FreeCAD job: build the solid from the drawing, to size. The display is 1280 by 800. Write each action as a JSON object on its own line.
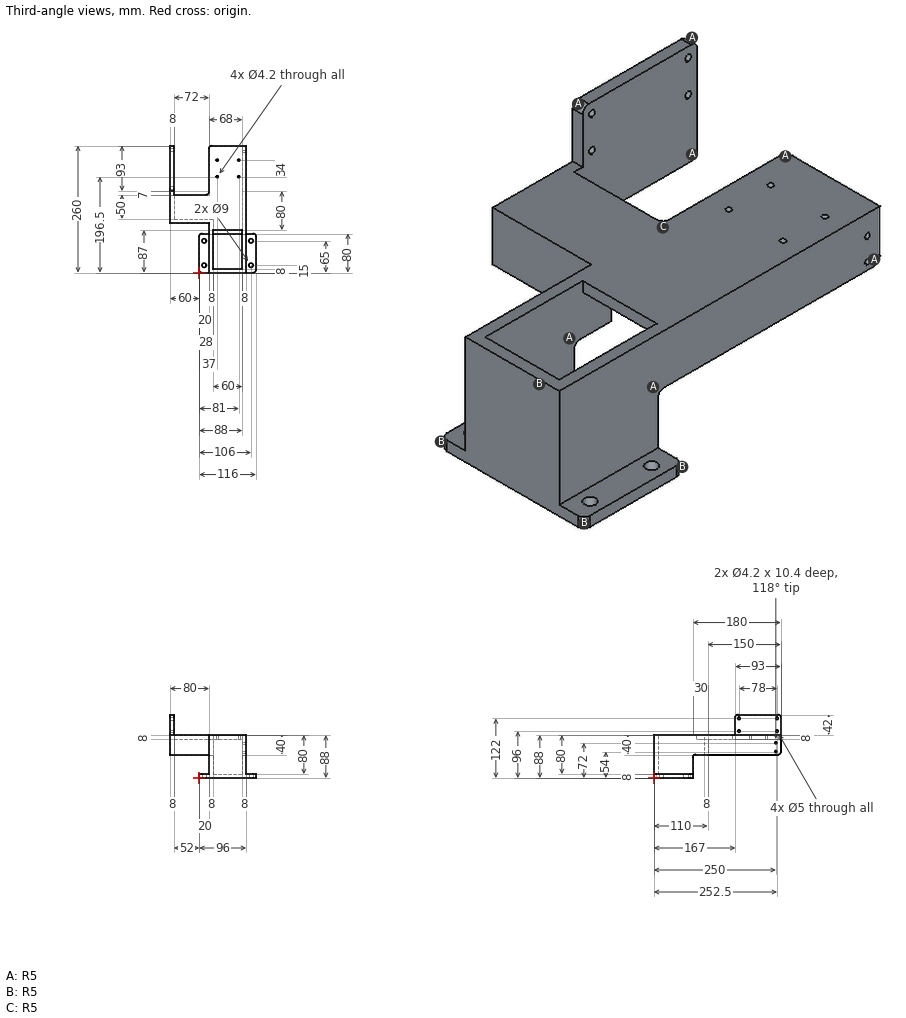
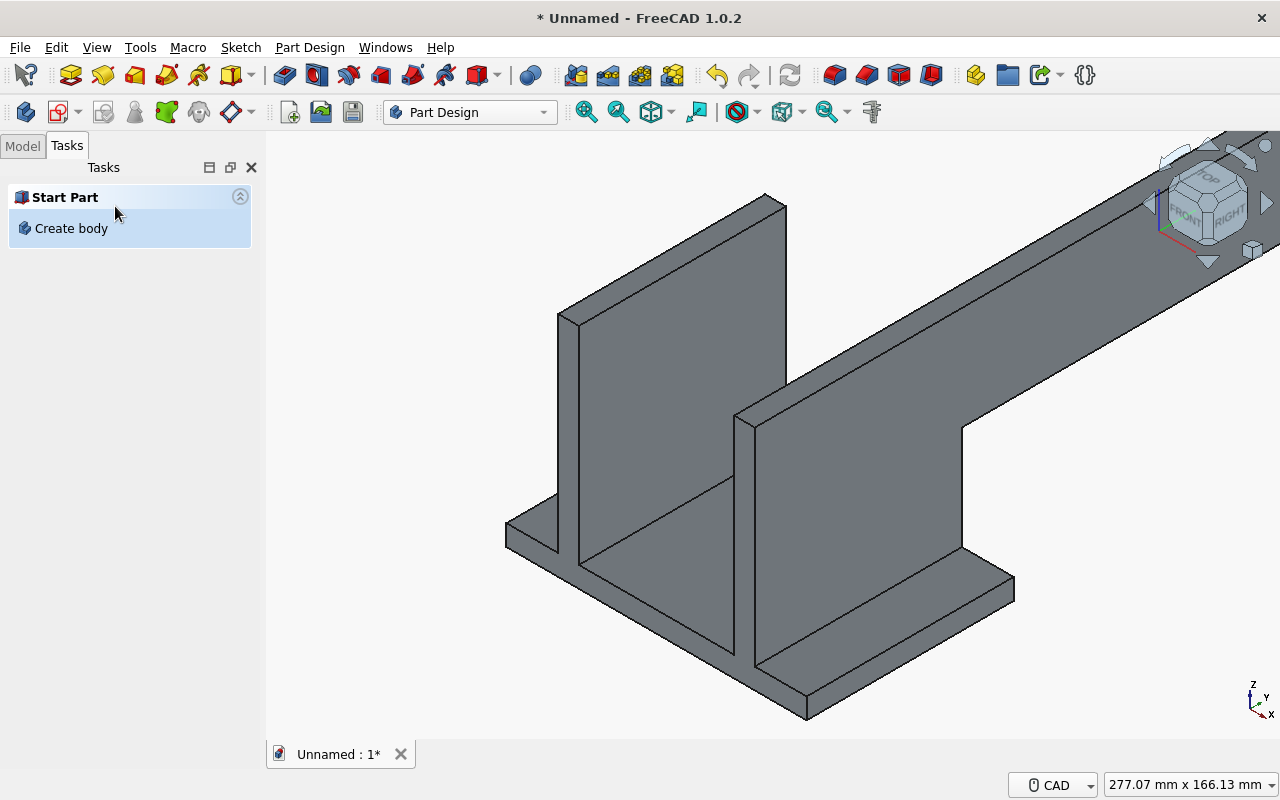
{"action": "left_click", "coordinate": [588, 112]}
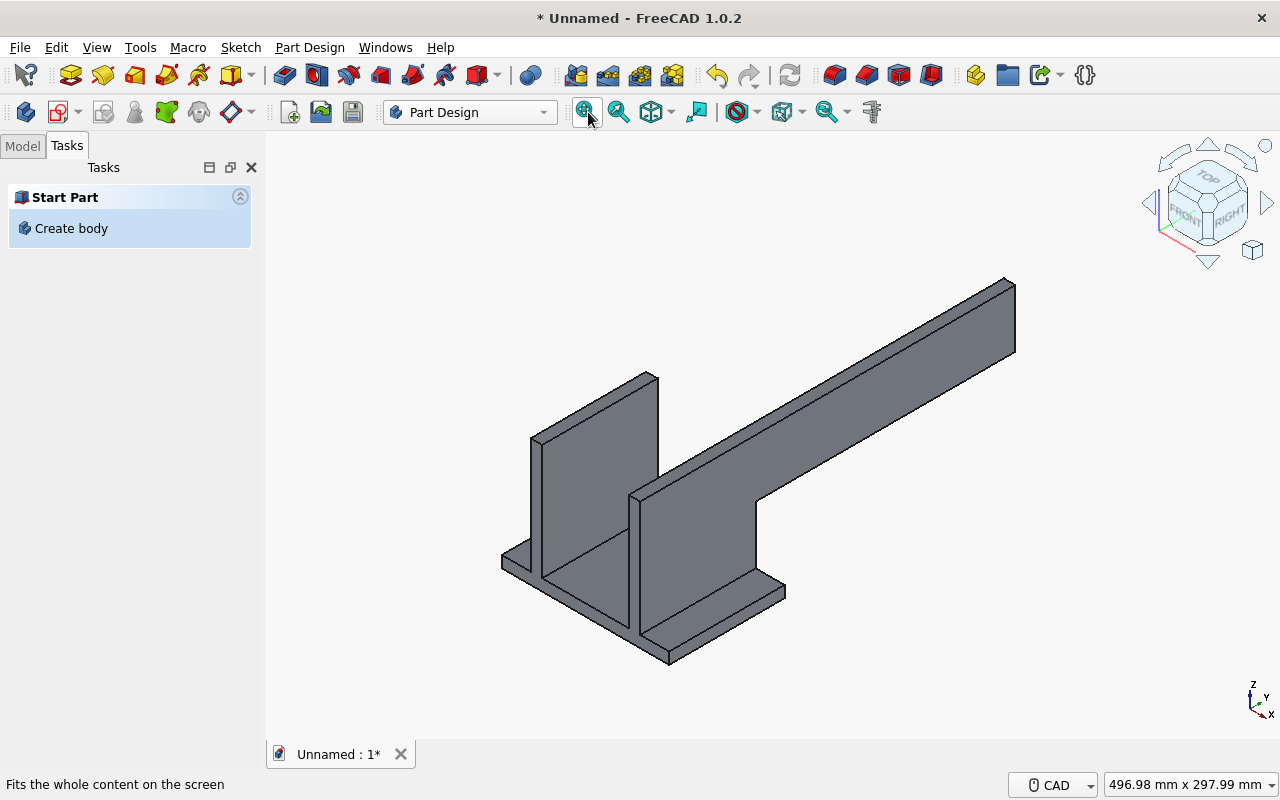
{"action": "key", "text": "2"}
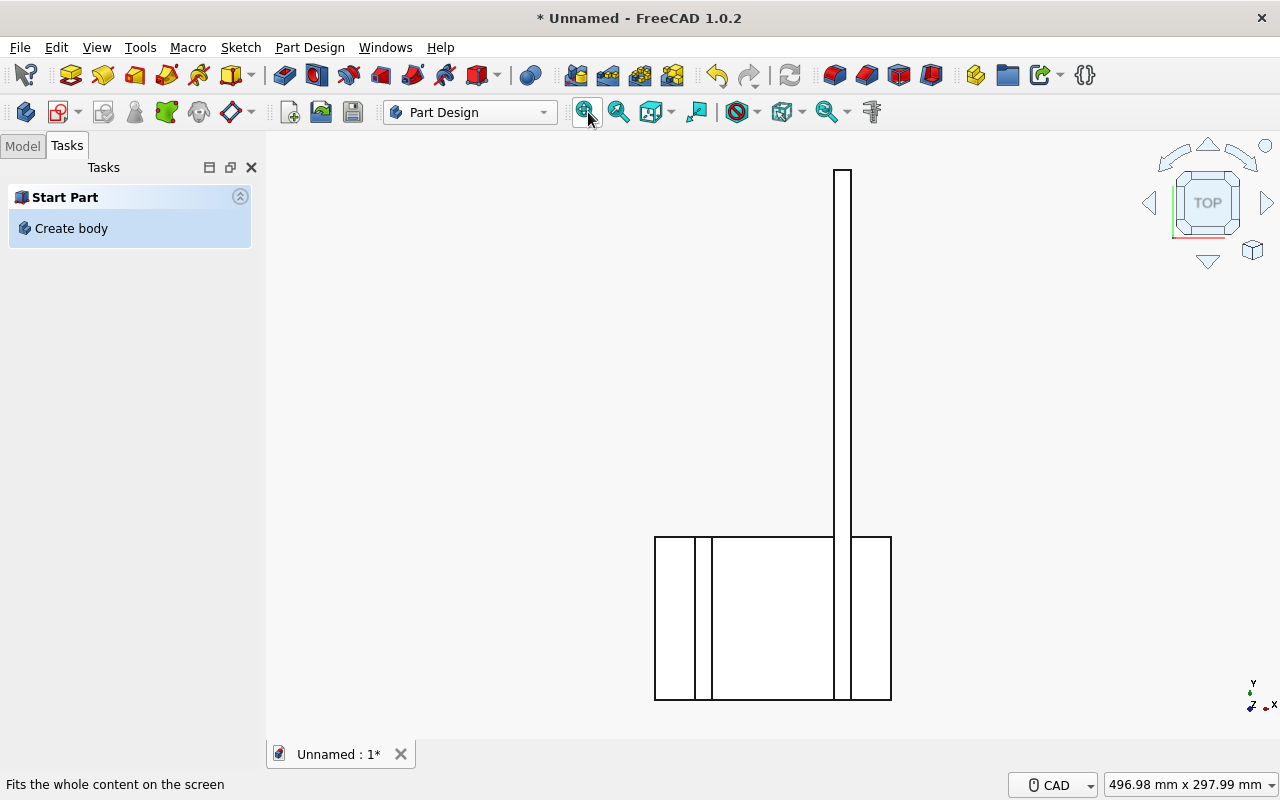
{"action": "left_click", "coordinate": [773, 618]}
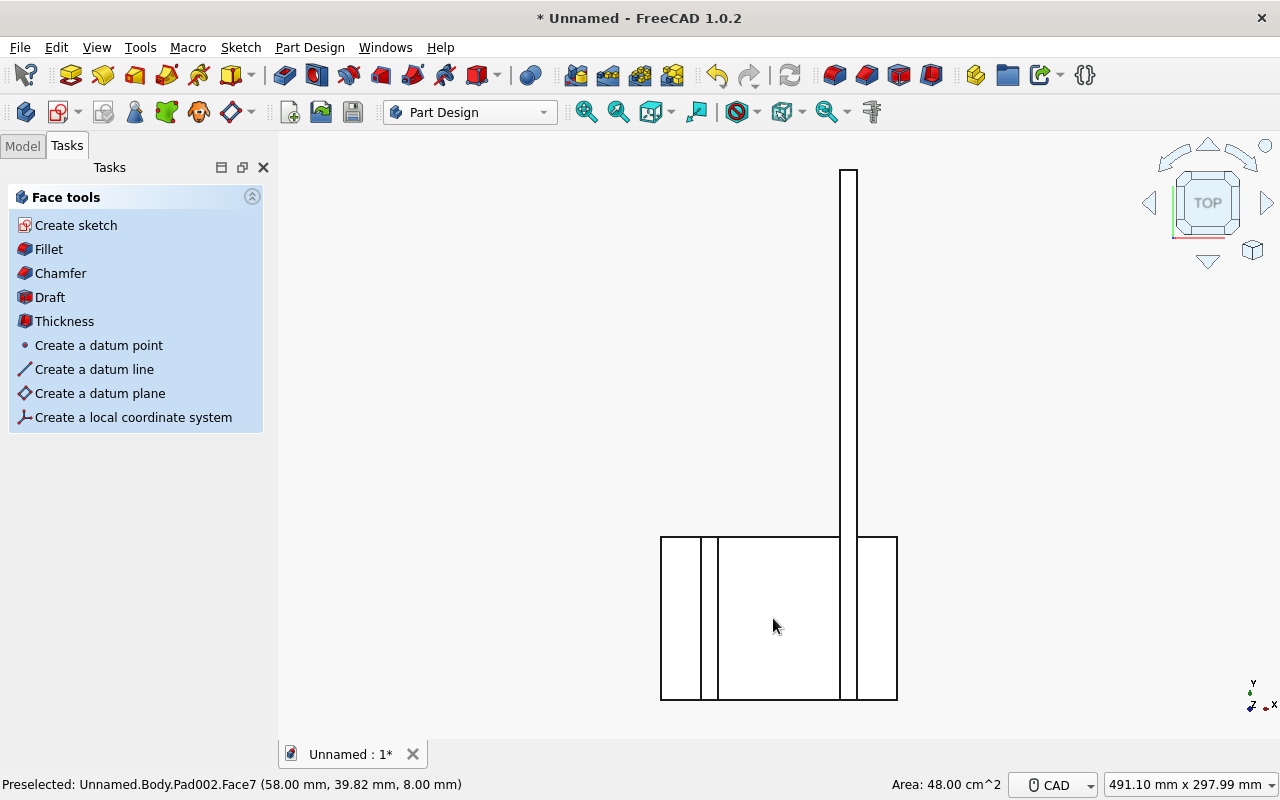
{"action": "left_click", "coordinate": [58, 112]}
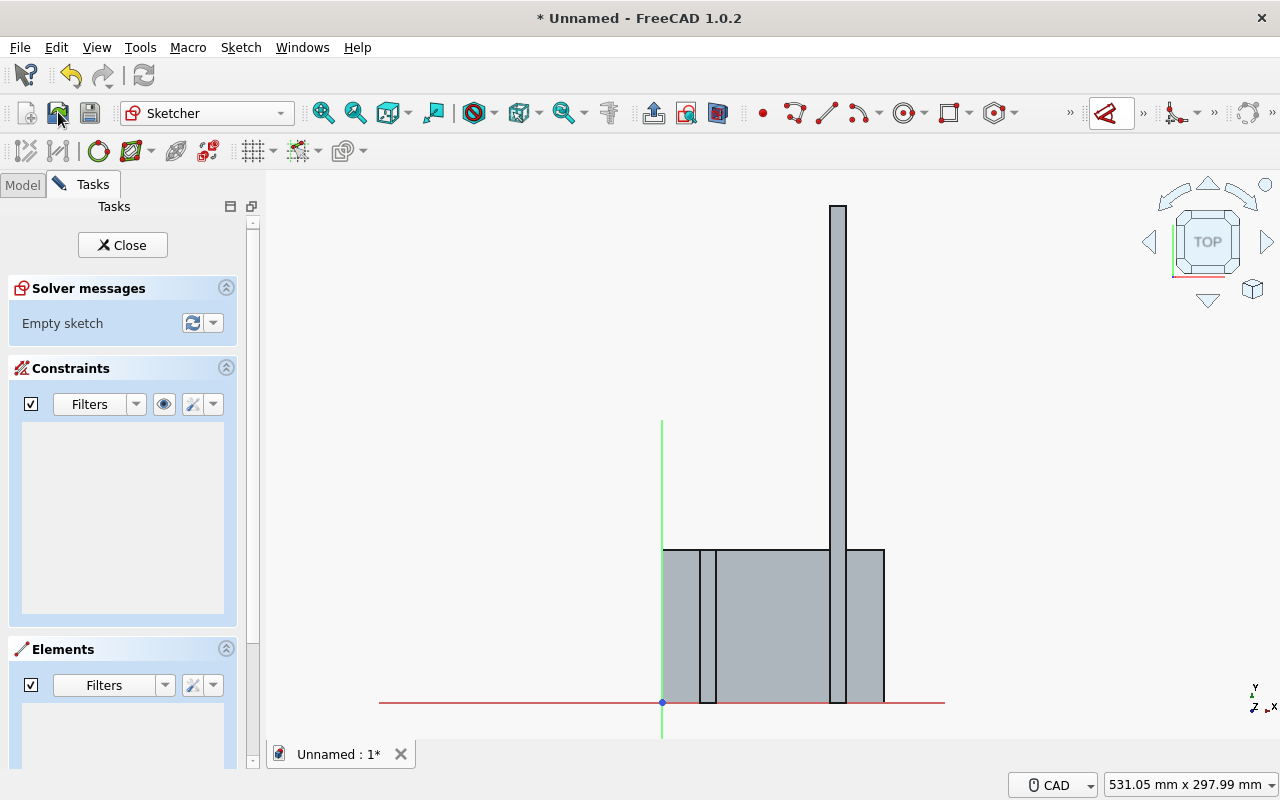
{"action": "scroll", "coordinate": [764, 711], "scroll_direction": "up", "scroll_amount": 6}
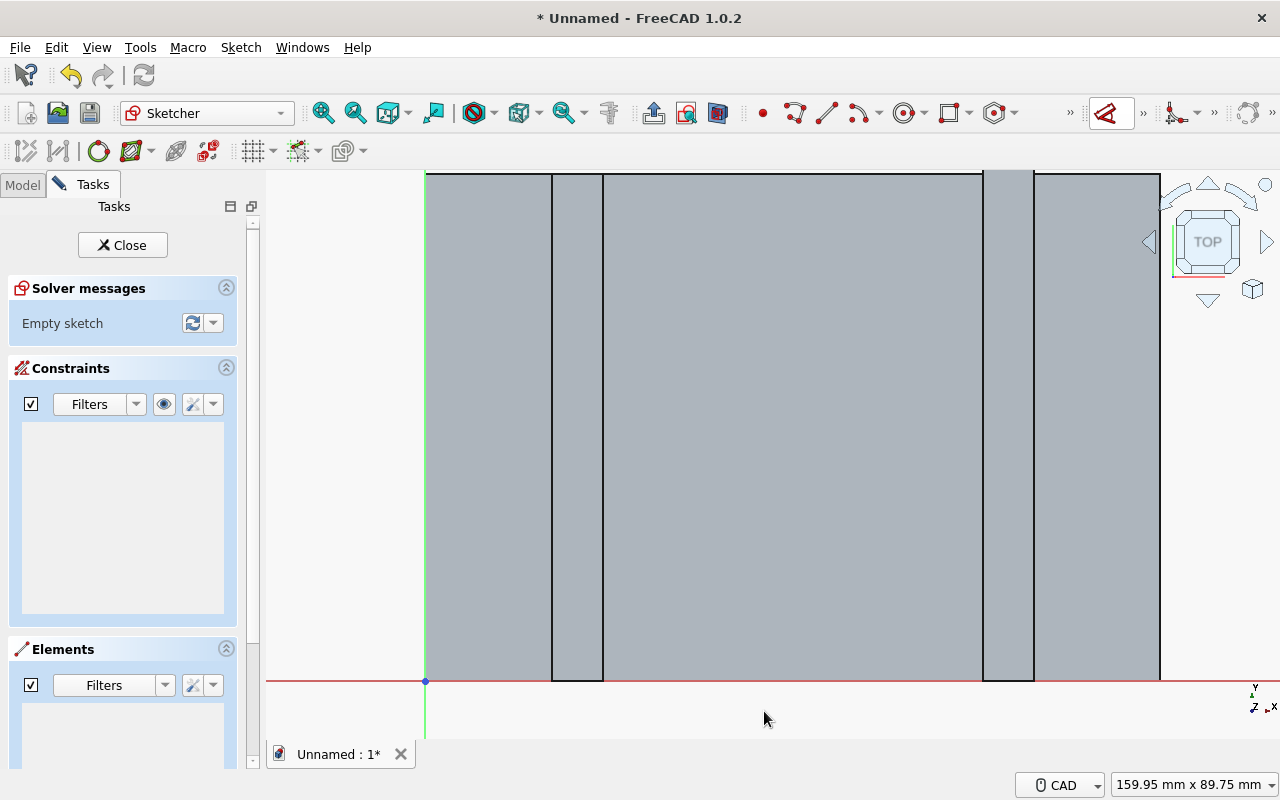
{"action": "left_click", "coordinate": [950, 114]}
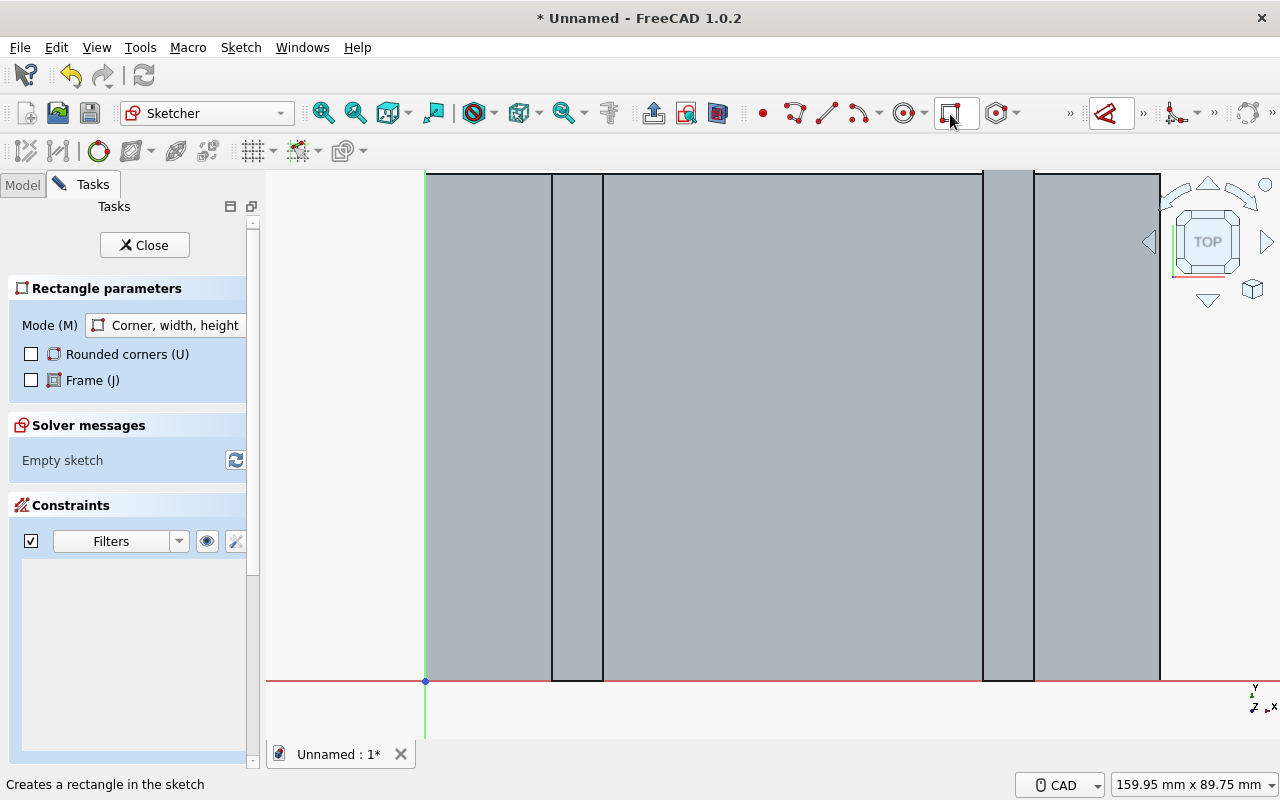
{"action": "left_click", "coordinate": [603, 631]}
{"action": "left_click", "coordinate": [983, 681]}
{"action": "key", "text": "Escape"}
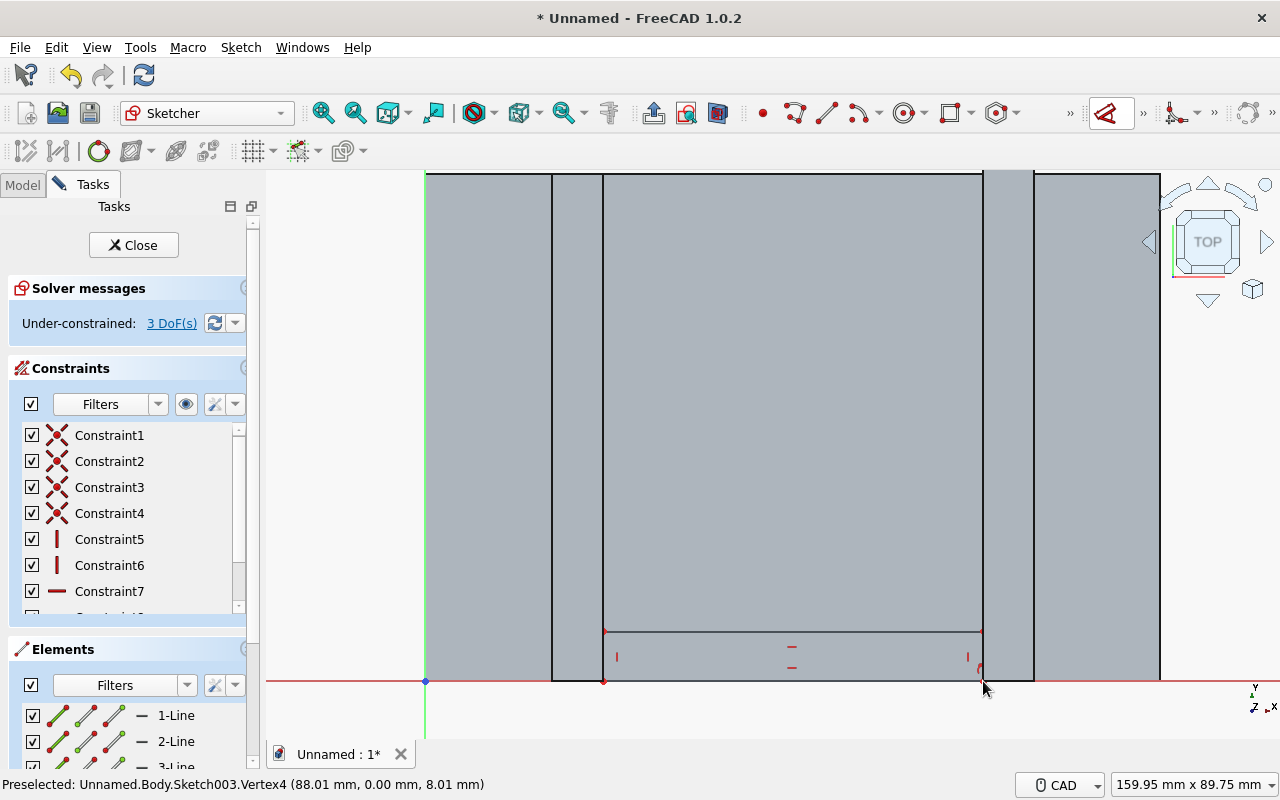
{"action": "left_click", "coordinate": [603, 647]}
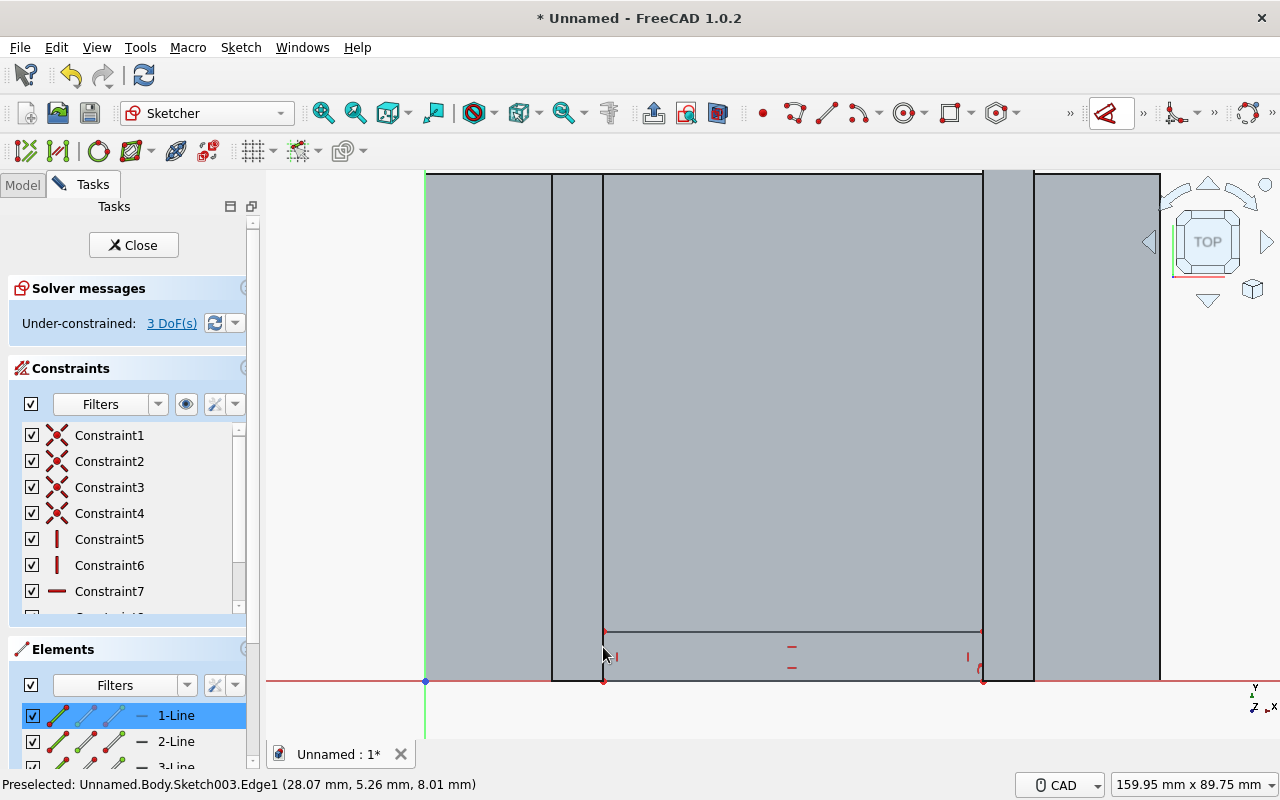
{"action": "left_click", "coordinate": [1128, 114]}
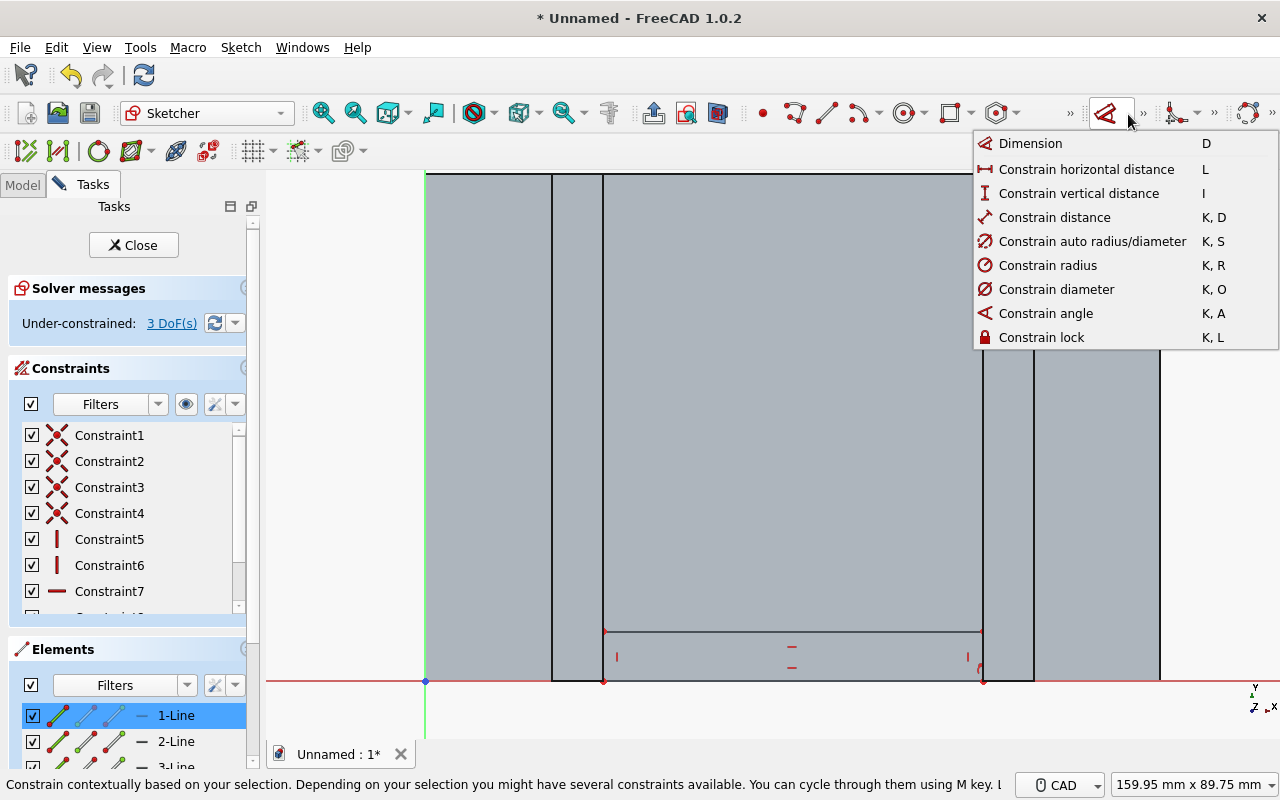
{"action": "left_click", "coordinate": [1126, 193]}